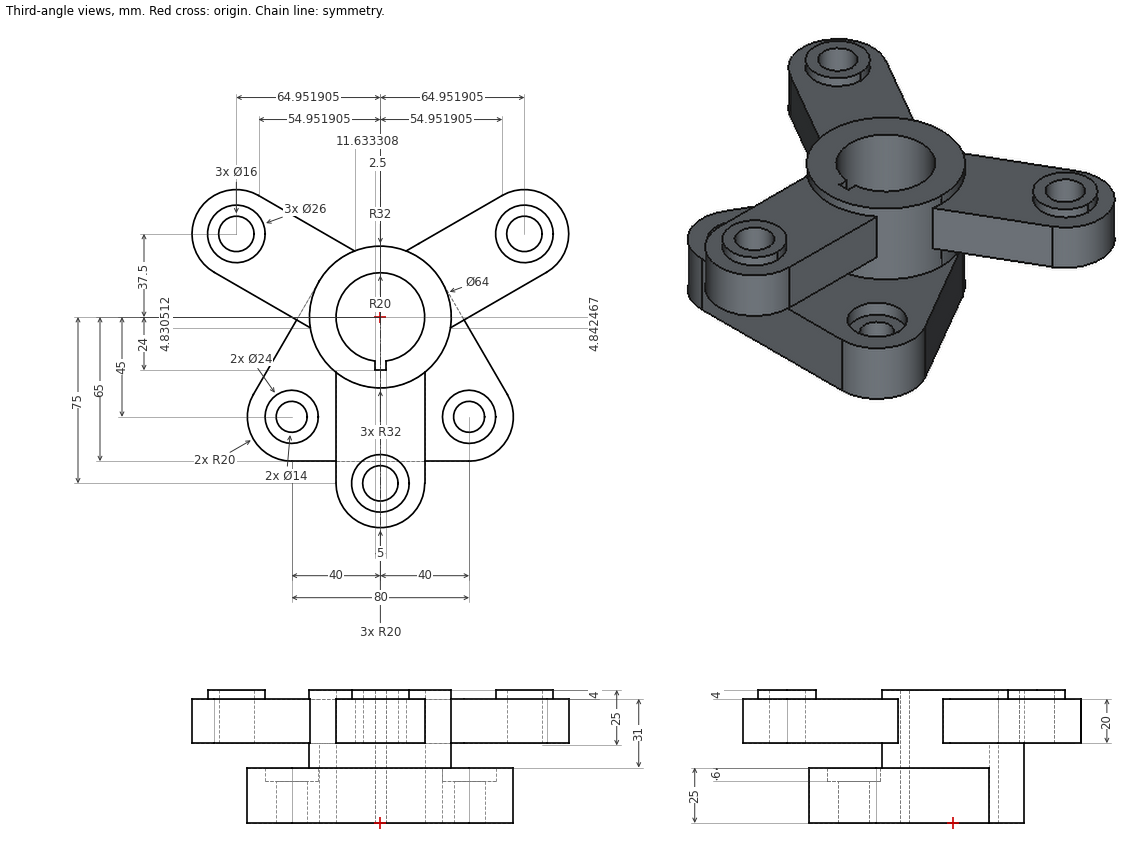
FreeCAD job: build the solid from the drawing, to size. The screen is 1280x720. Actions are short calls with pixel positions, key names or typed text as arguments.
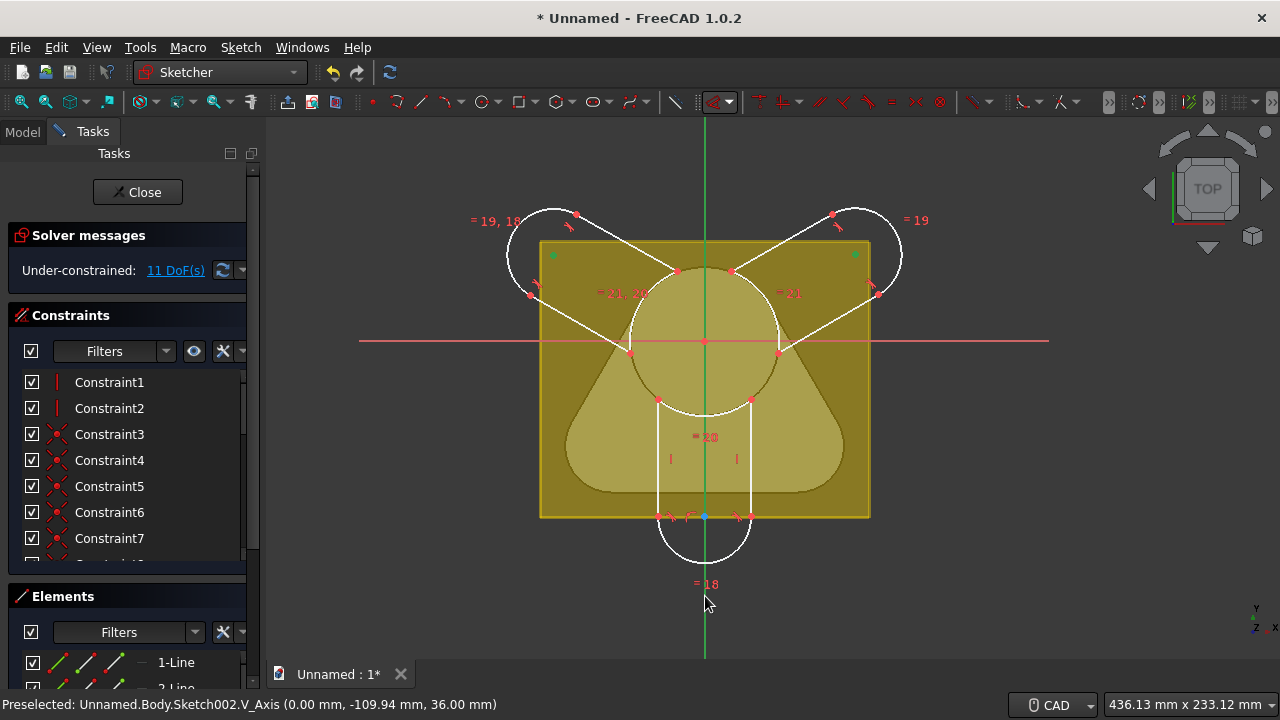
key(s)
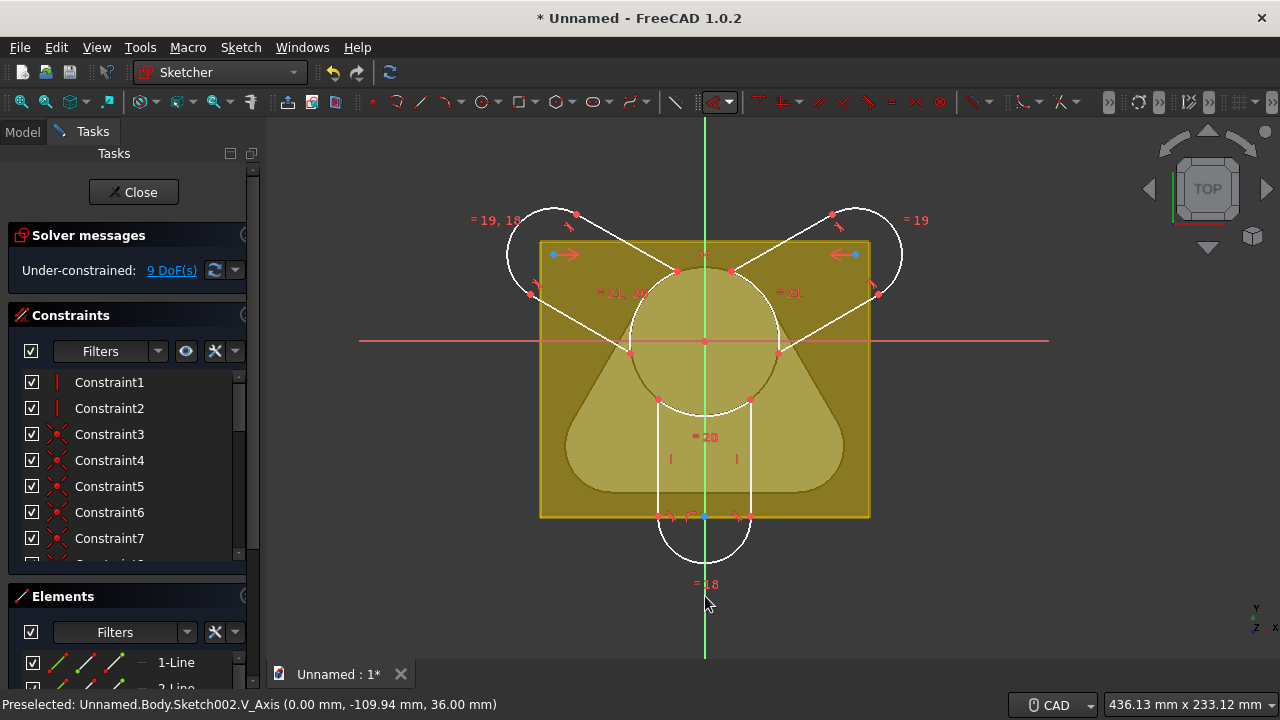
click(677, 554)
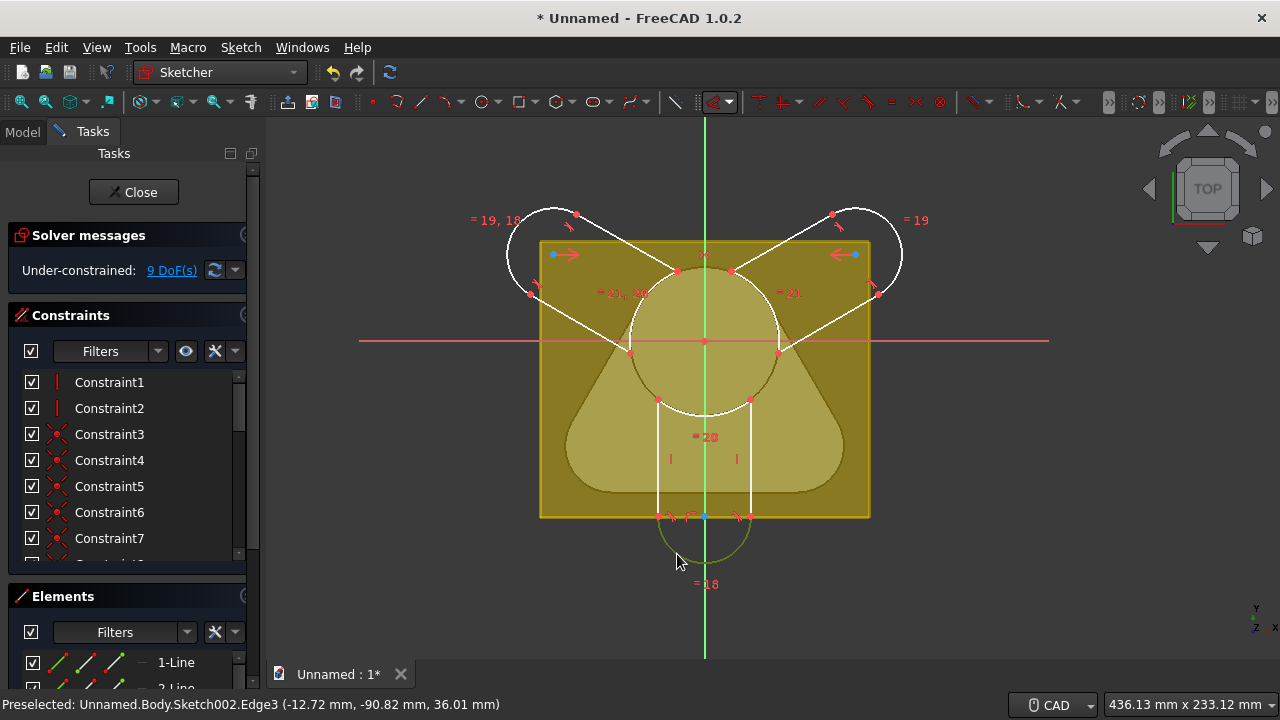
click(732, 102)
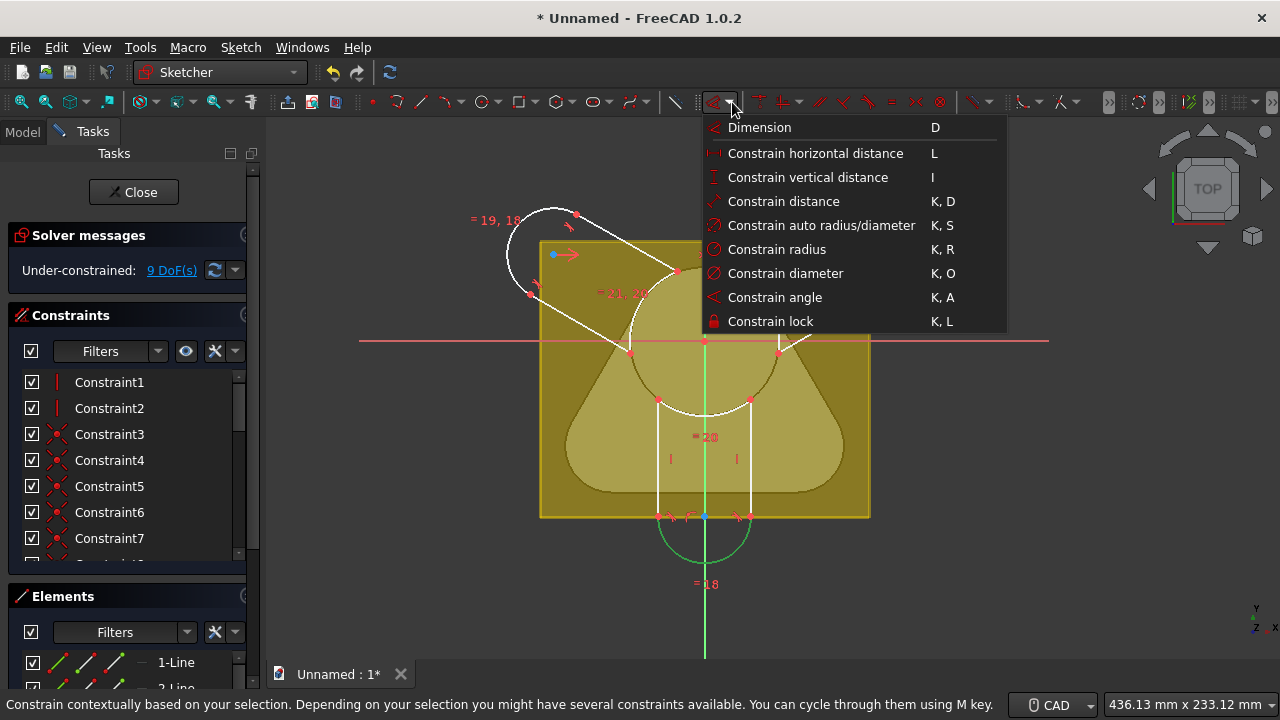
click(855, 249)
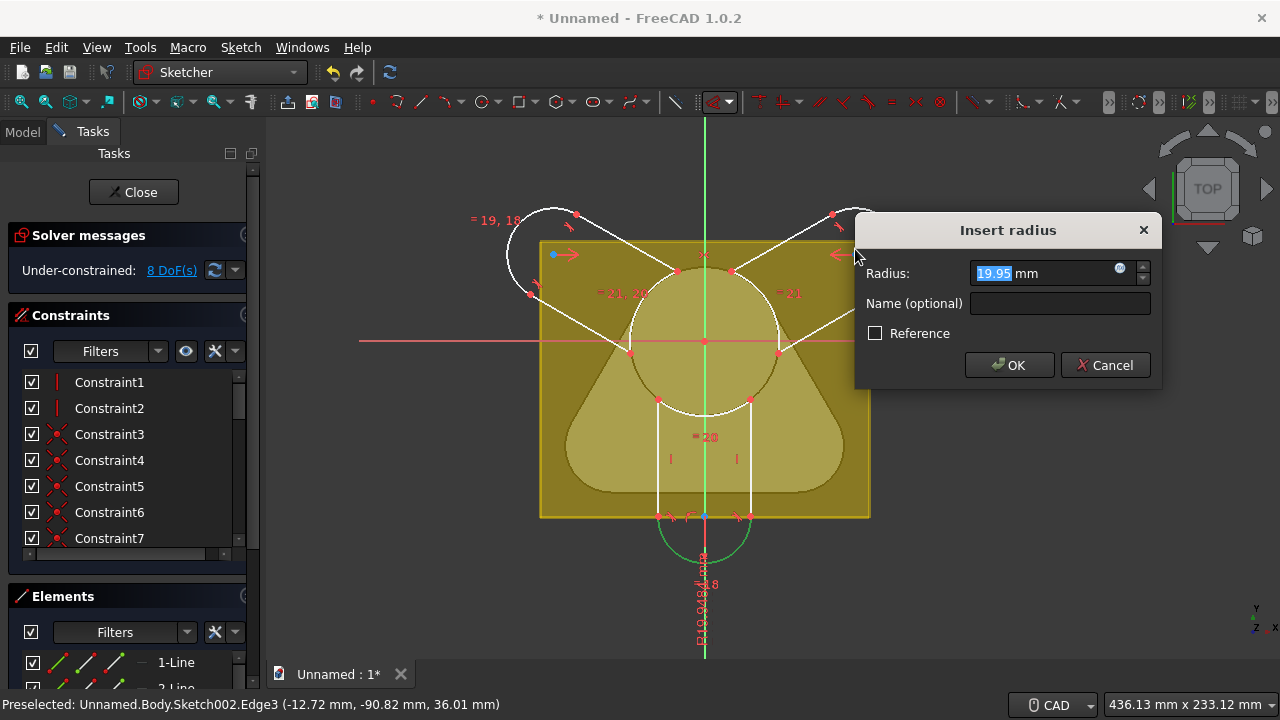
text(20)
key(Return)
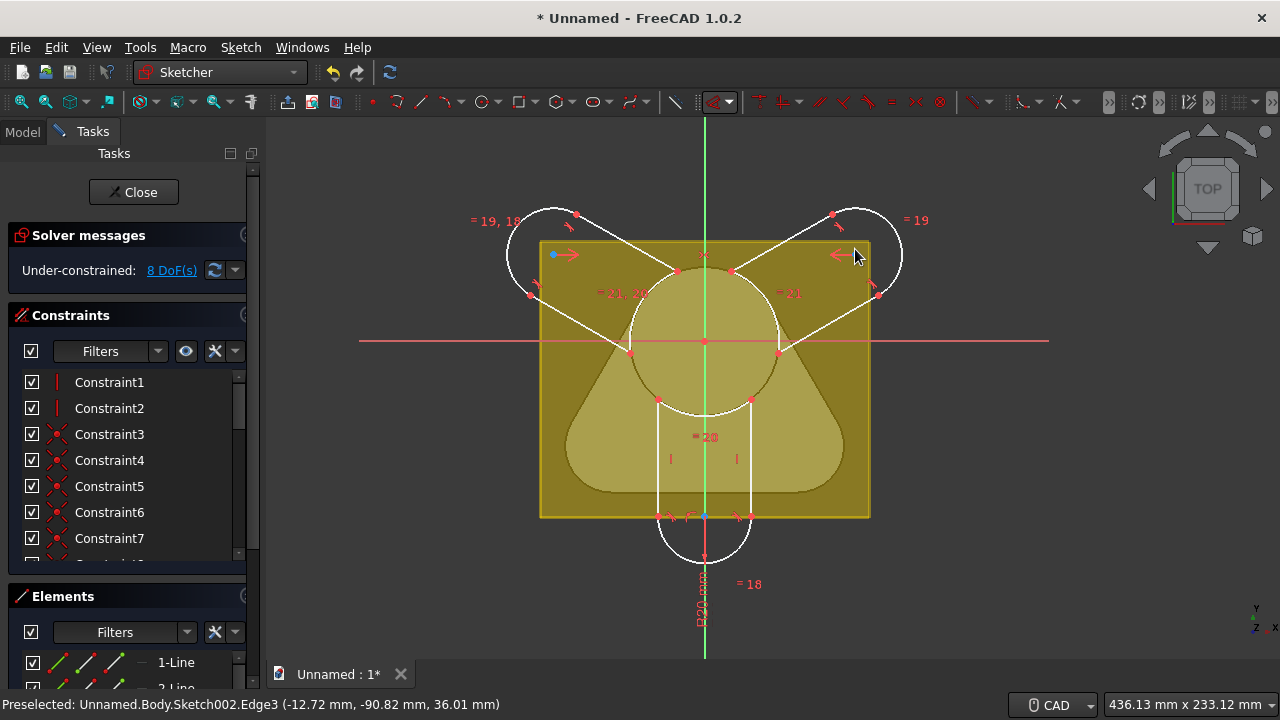
click(685, 414)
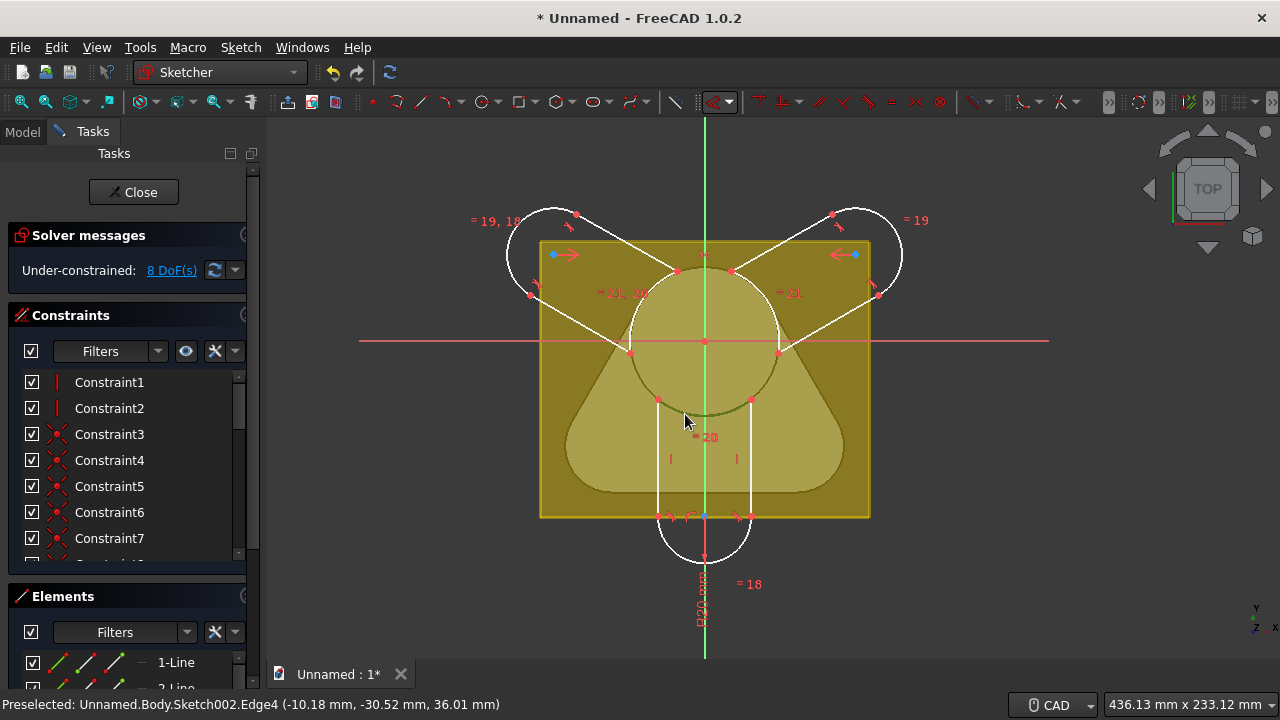
key(k)
key(r)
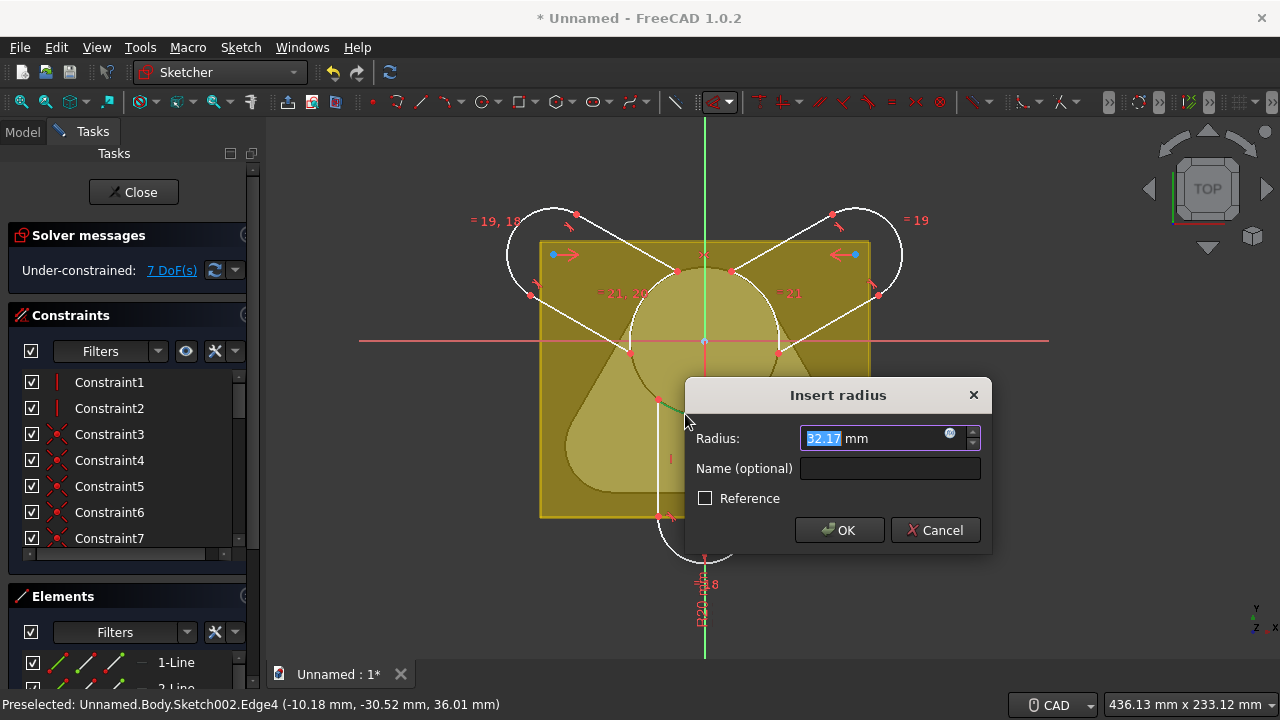
text(32)
key(Return)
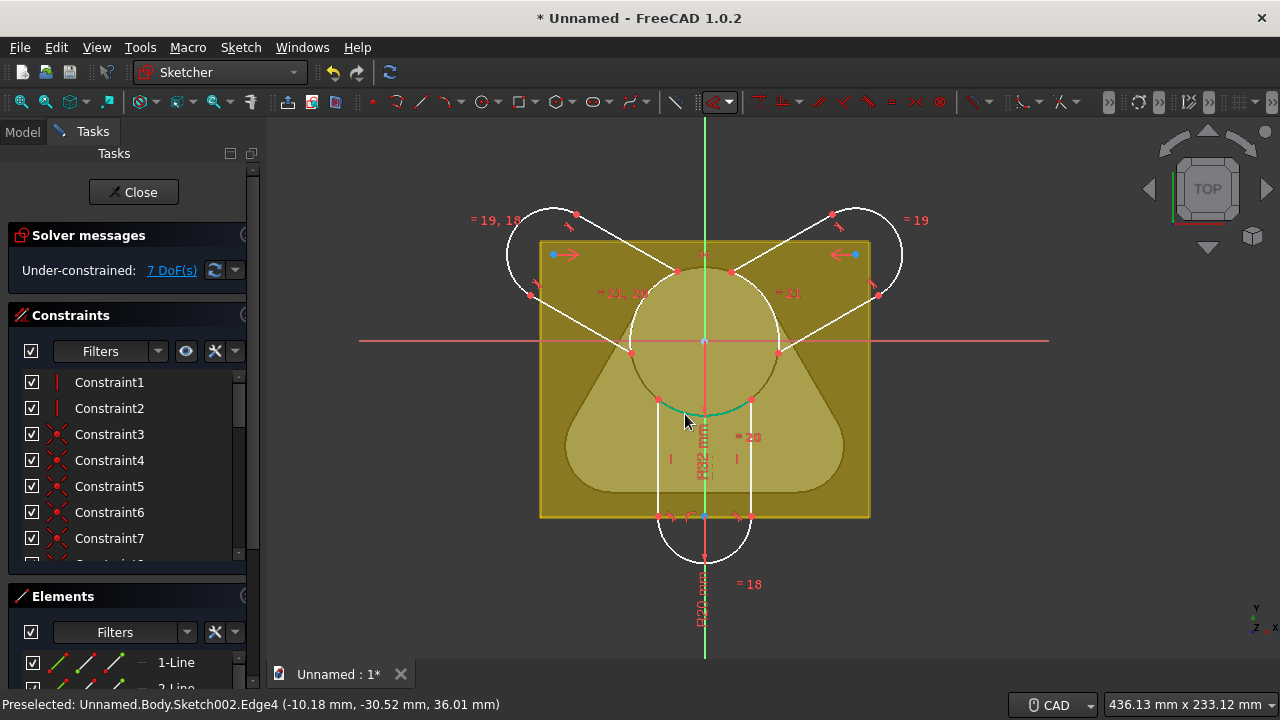
click(658, 517)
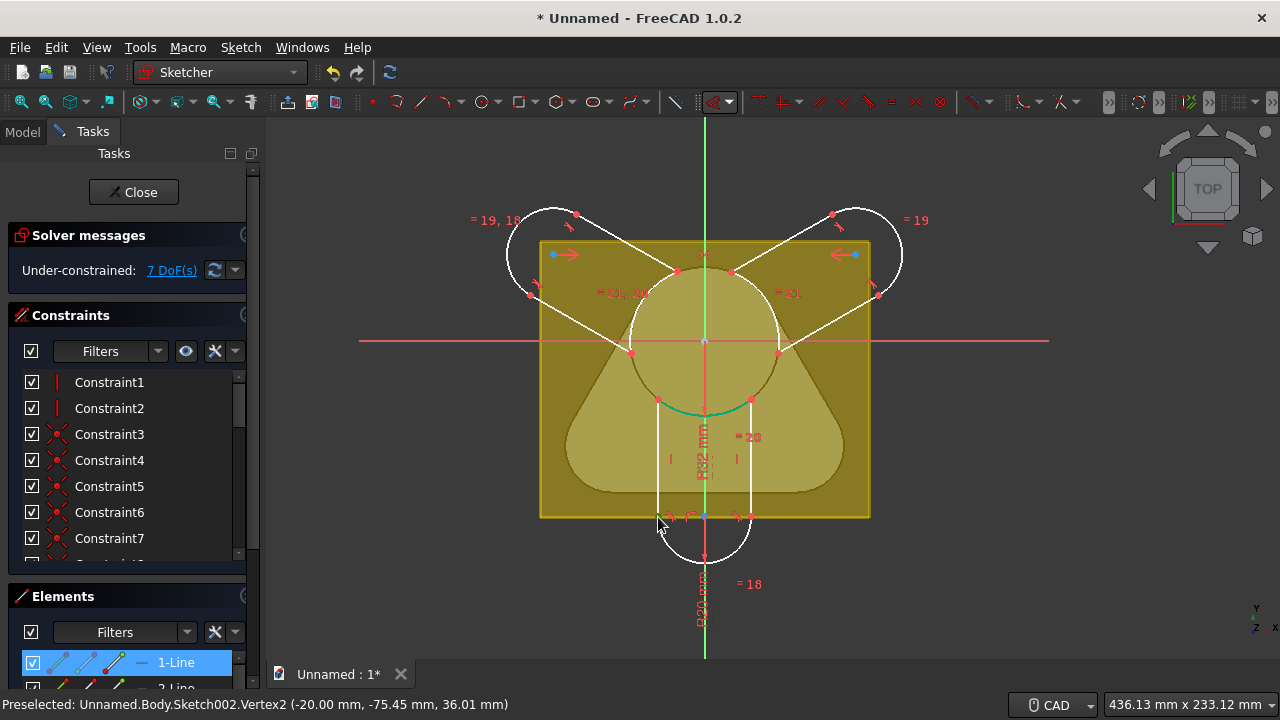
key(i)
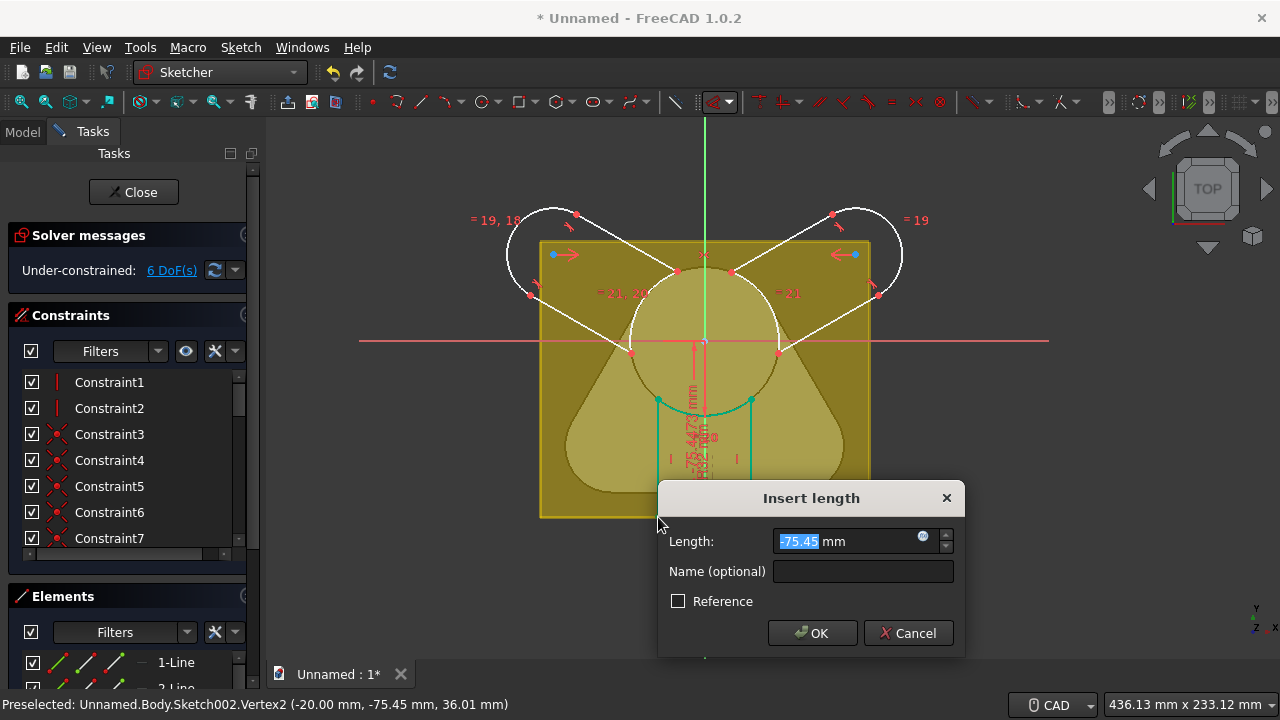
text(-75)
key(Return)